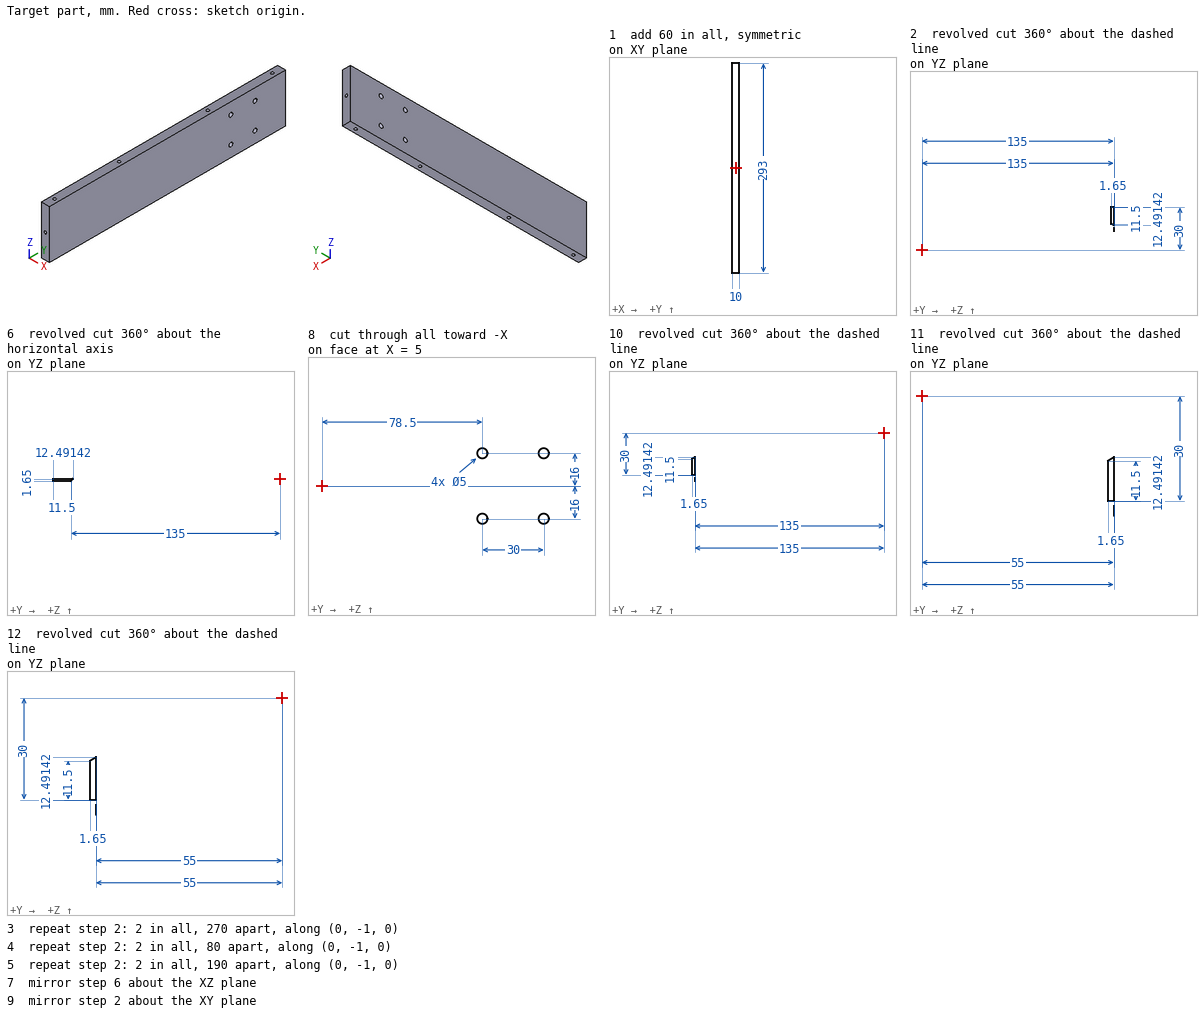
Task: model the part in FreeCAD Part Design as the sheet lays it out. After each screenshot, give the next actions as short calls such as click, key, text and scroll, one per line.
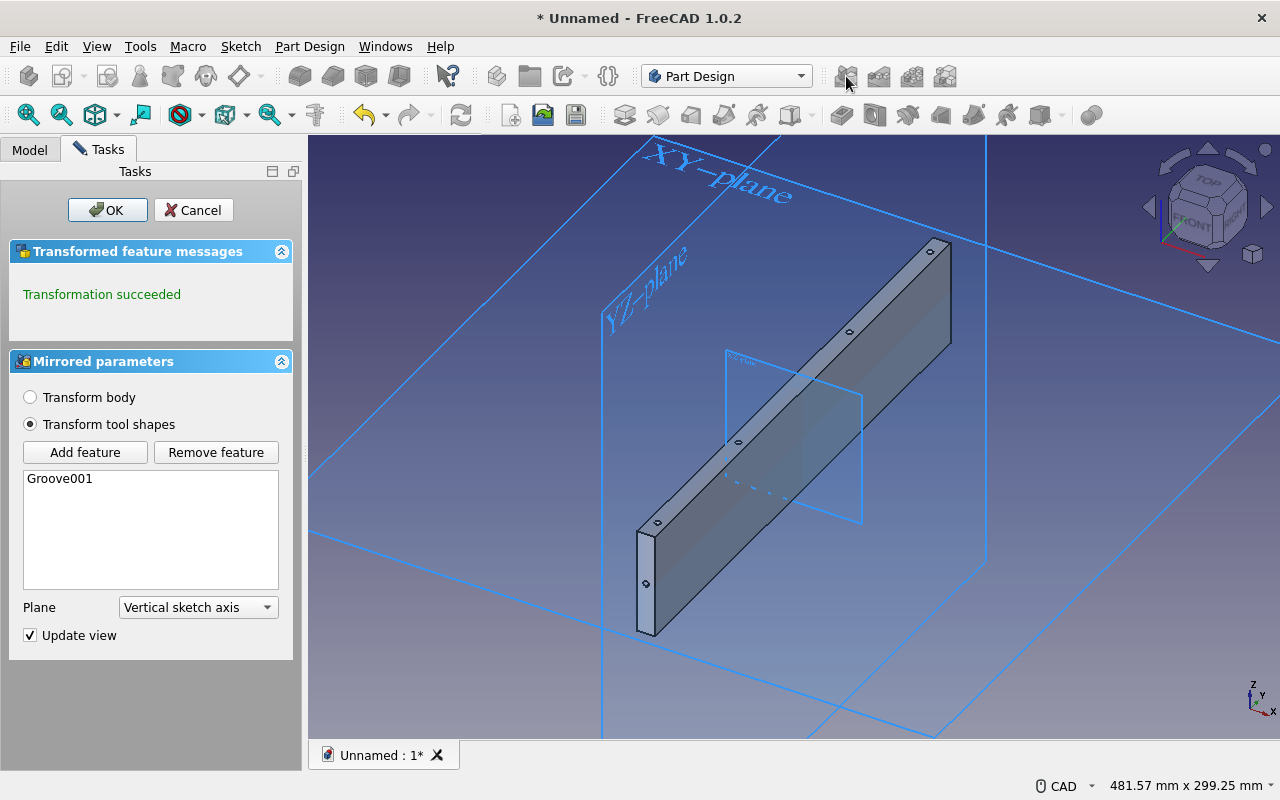
click(199, 608)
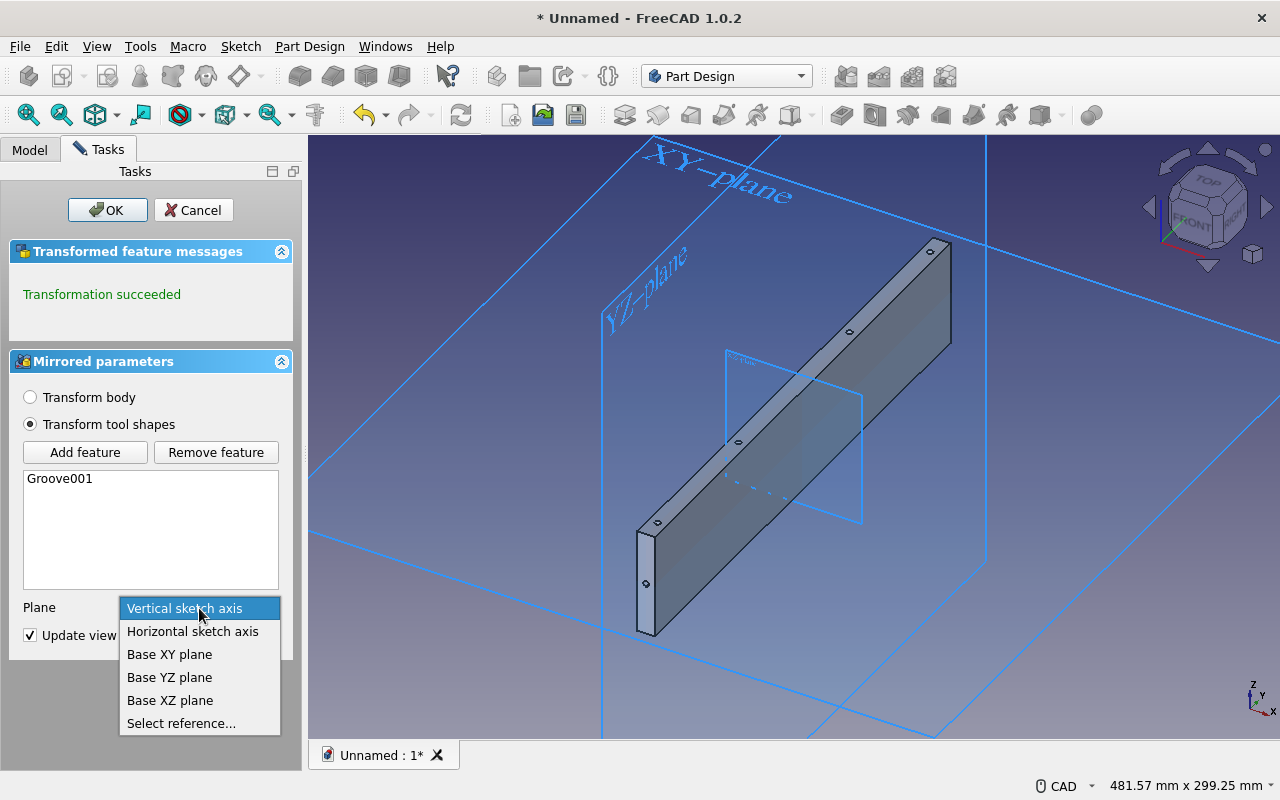
click(198, 700)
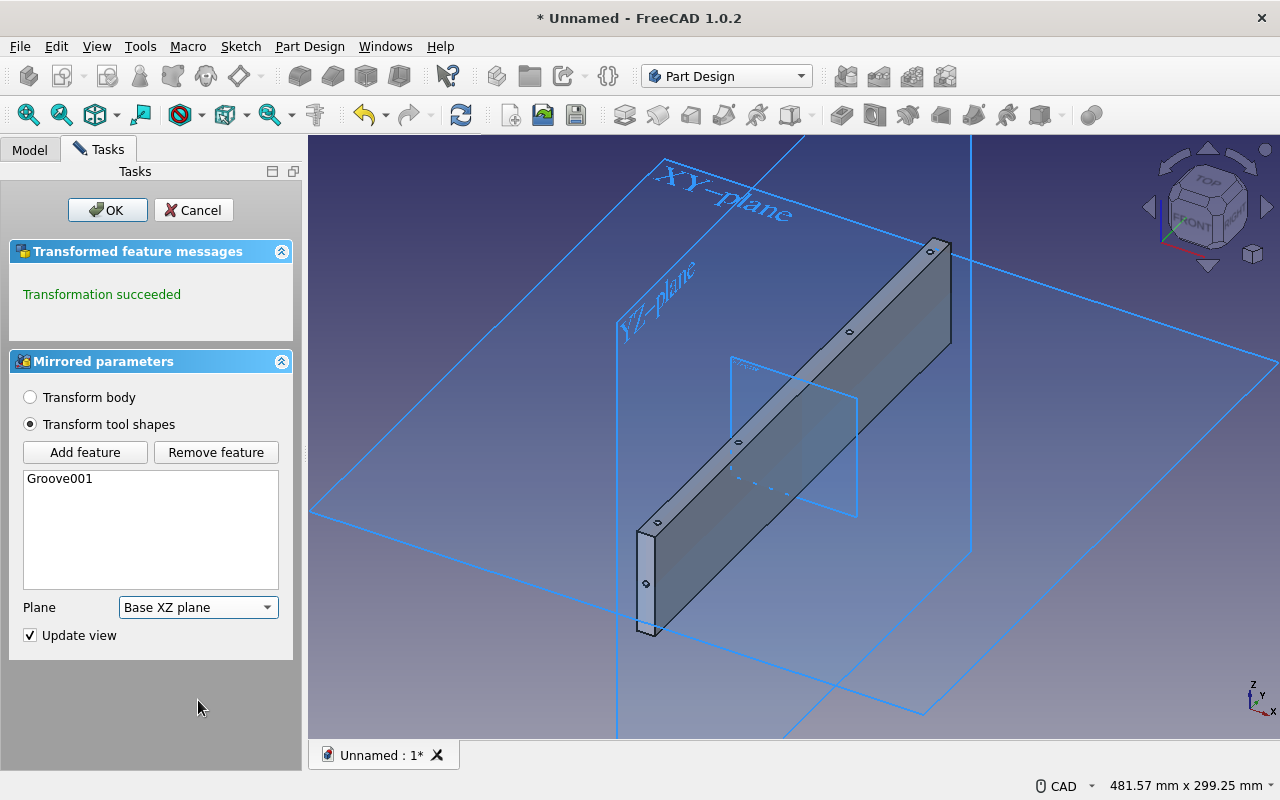
click(108, 210)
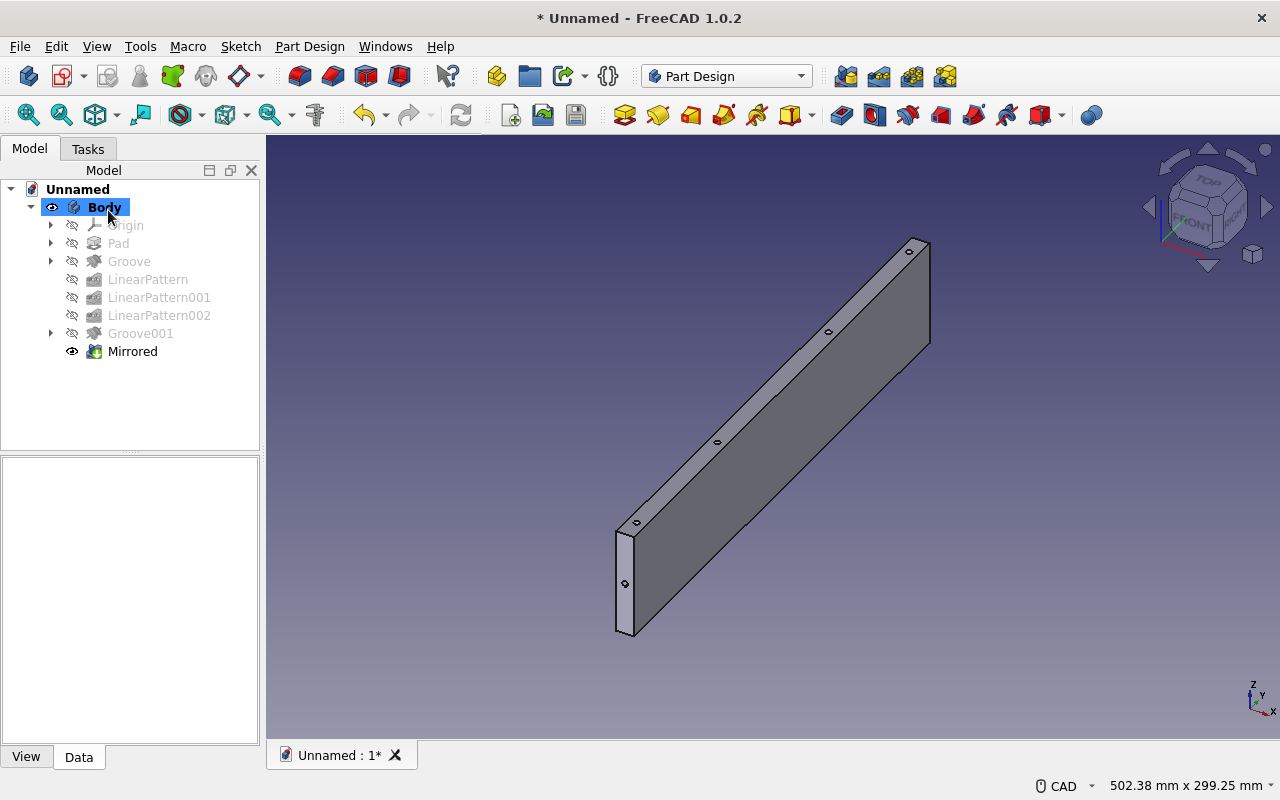
click(866, 355)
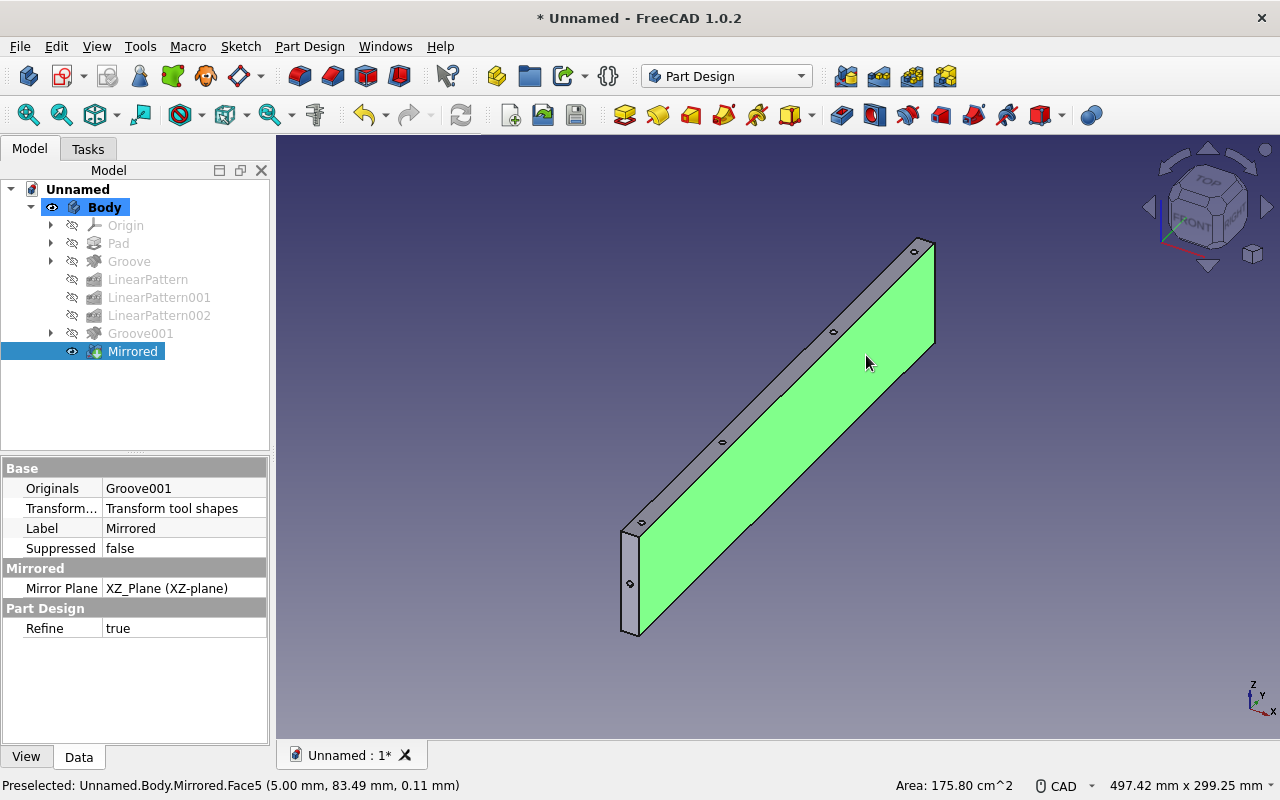
click(62, 76)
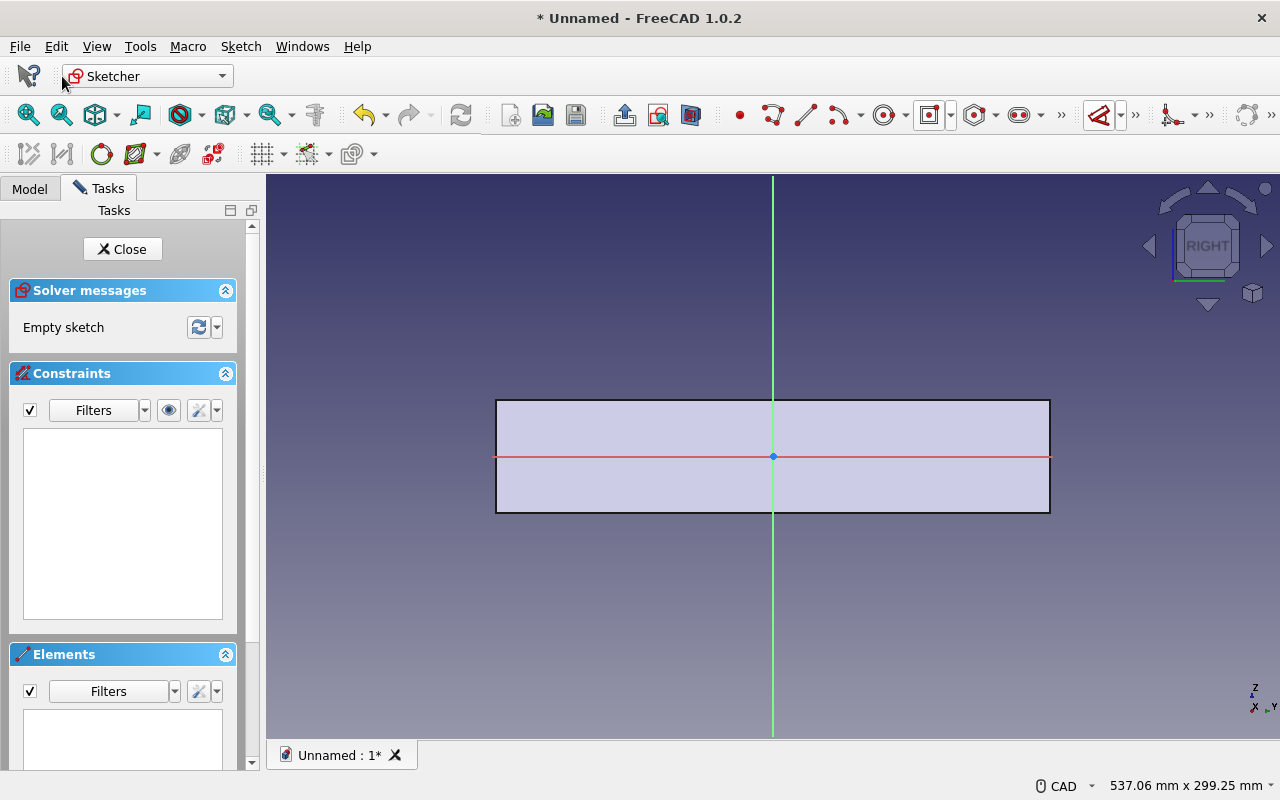
scroll(1012, 456, up, 8)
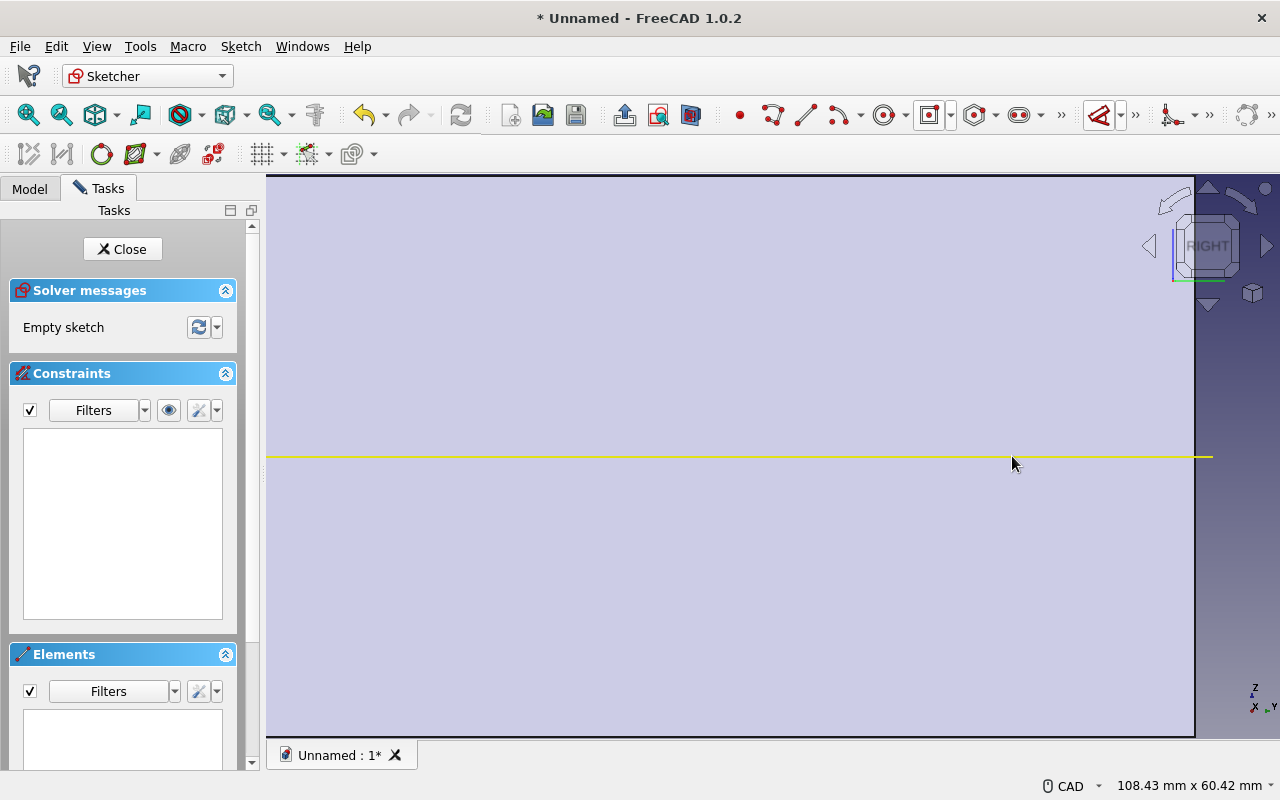
click(884, 116)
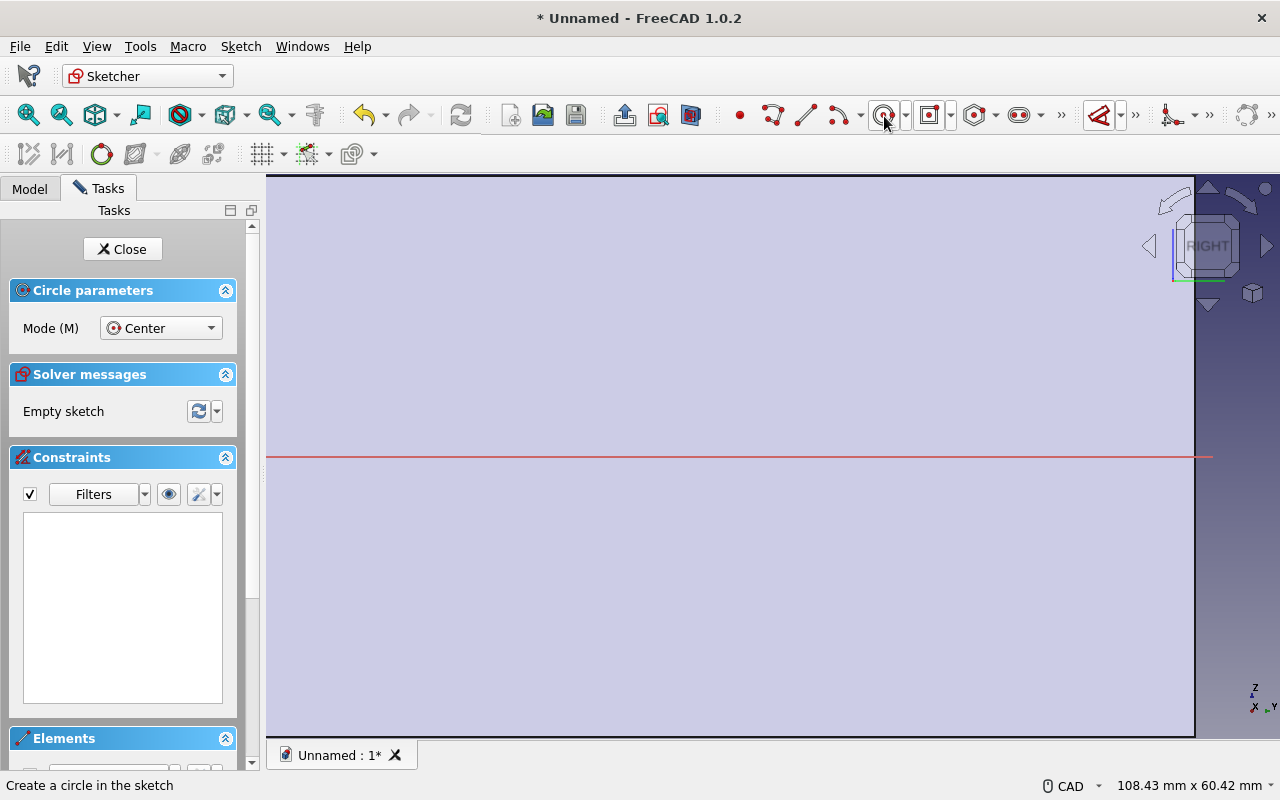
click(559, 307)
move(576, 290)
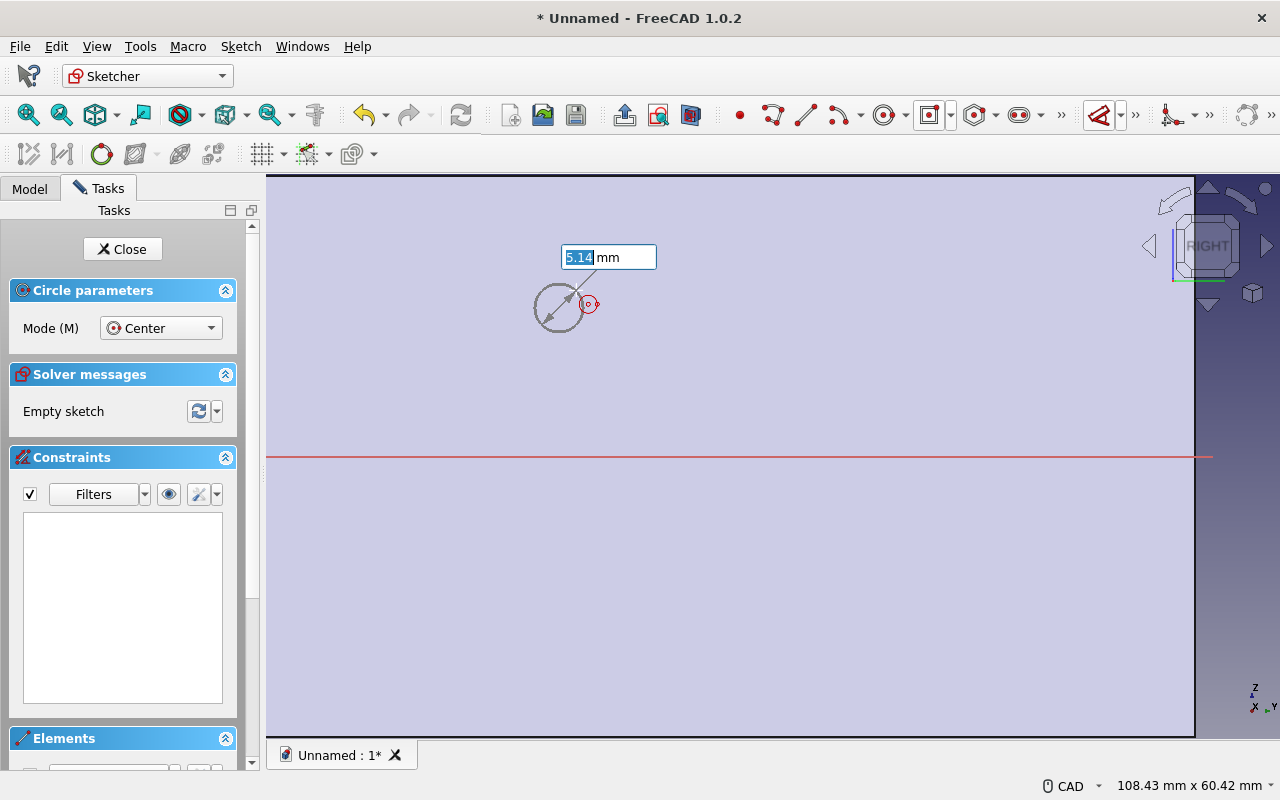
text(5)
key(Return)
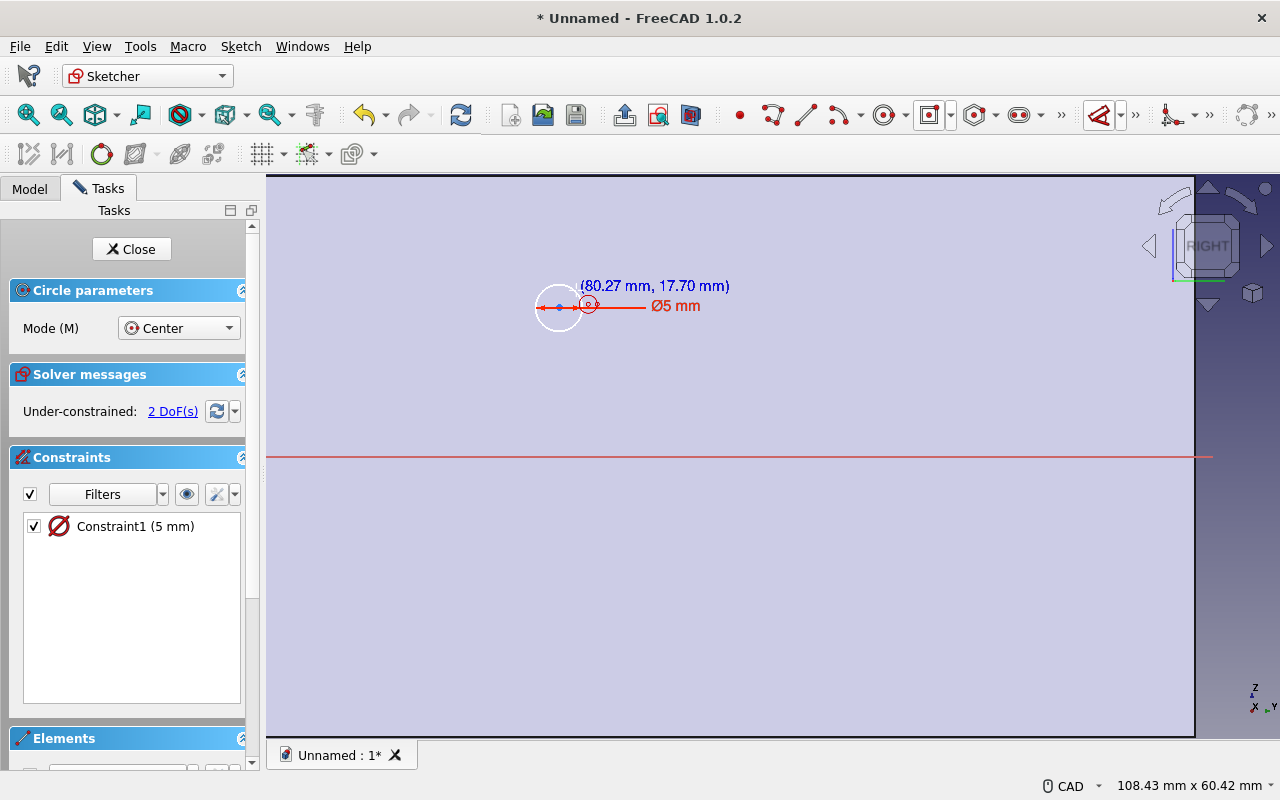
click(559, 606)
move(576, 590)